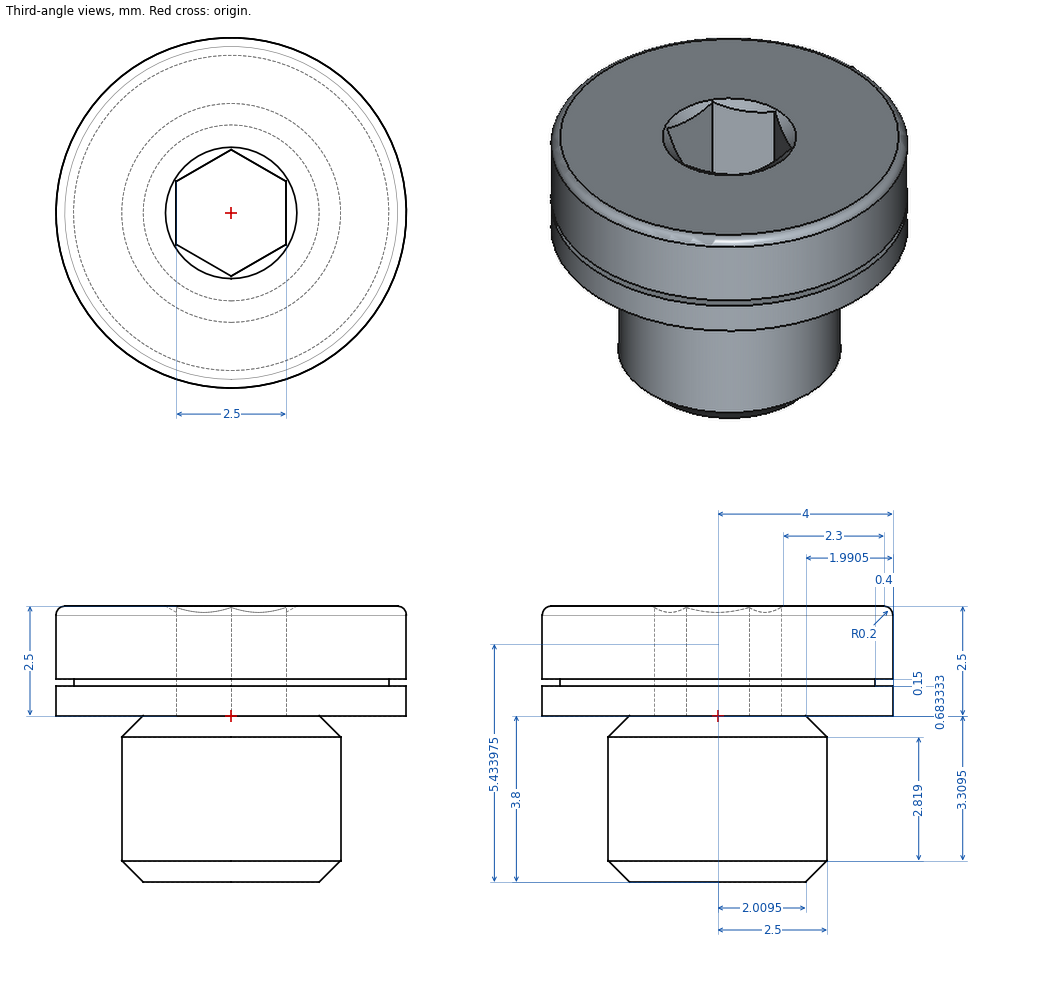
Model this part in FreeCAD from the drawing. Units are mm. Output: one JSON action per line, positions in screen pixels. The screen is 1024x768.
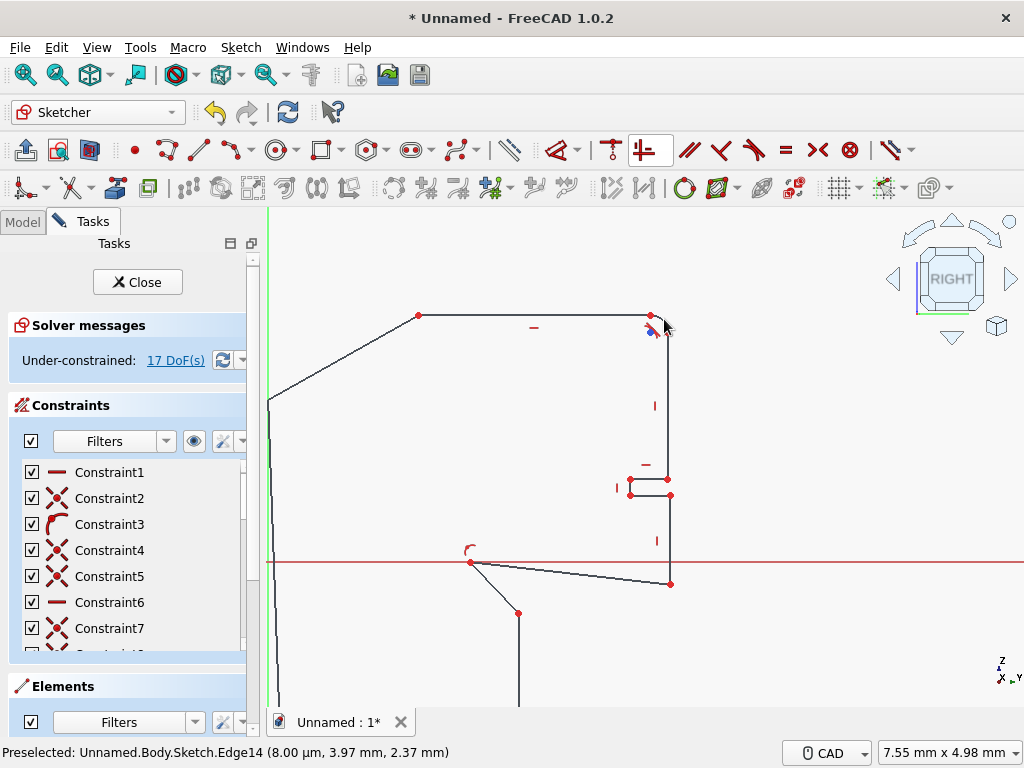
{"action": "scroll", "coordinate": [664, 318], "scroll_direction": "down", "scroll_amount": 4}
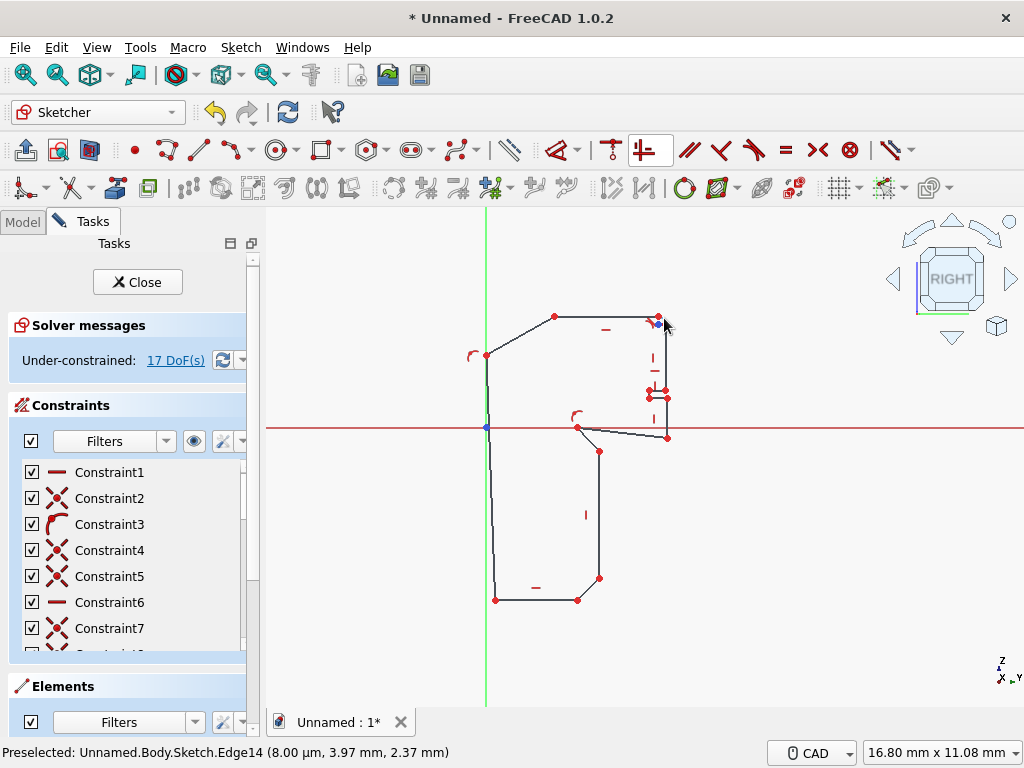
{"action": "scroll", "coordinate": [493, 527], "scroll_direction": "up", "scroll_amount": 5}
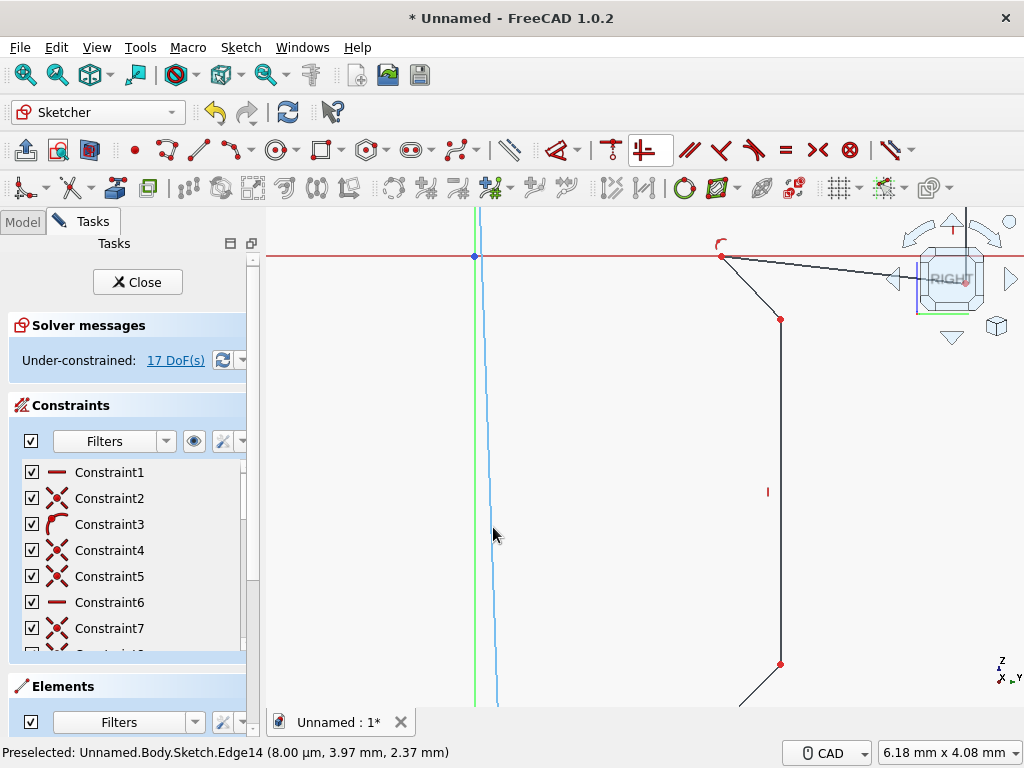
{"action": "left_click", "coordinate": [491, 525]}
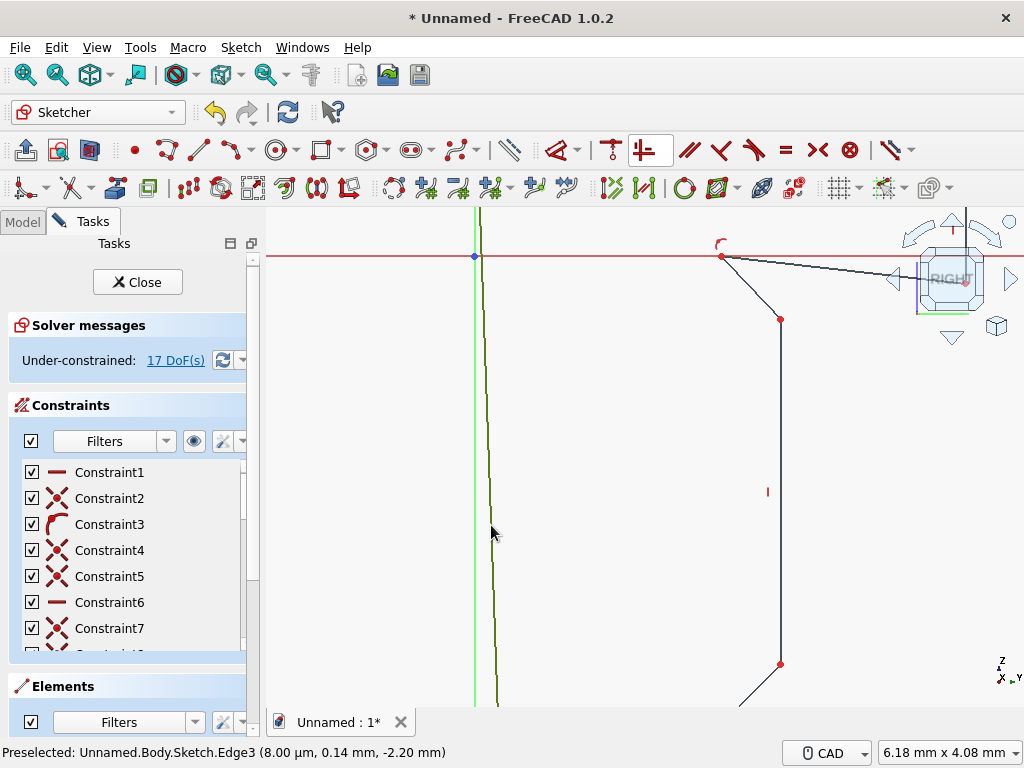
{"action": "left_click", "coordinate": [668, 150]}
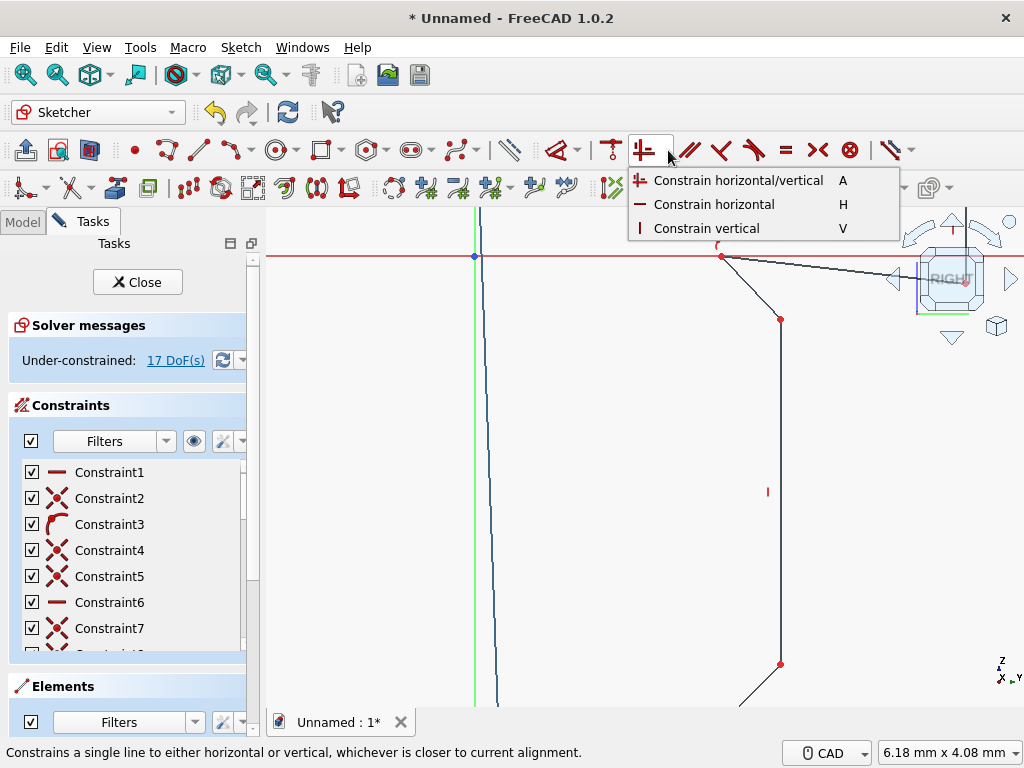
{"action": "left_click", "coordinate": [764, 228]}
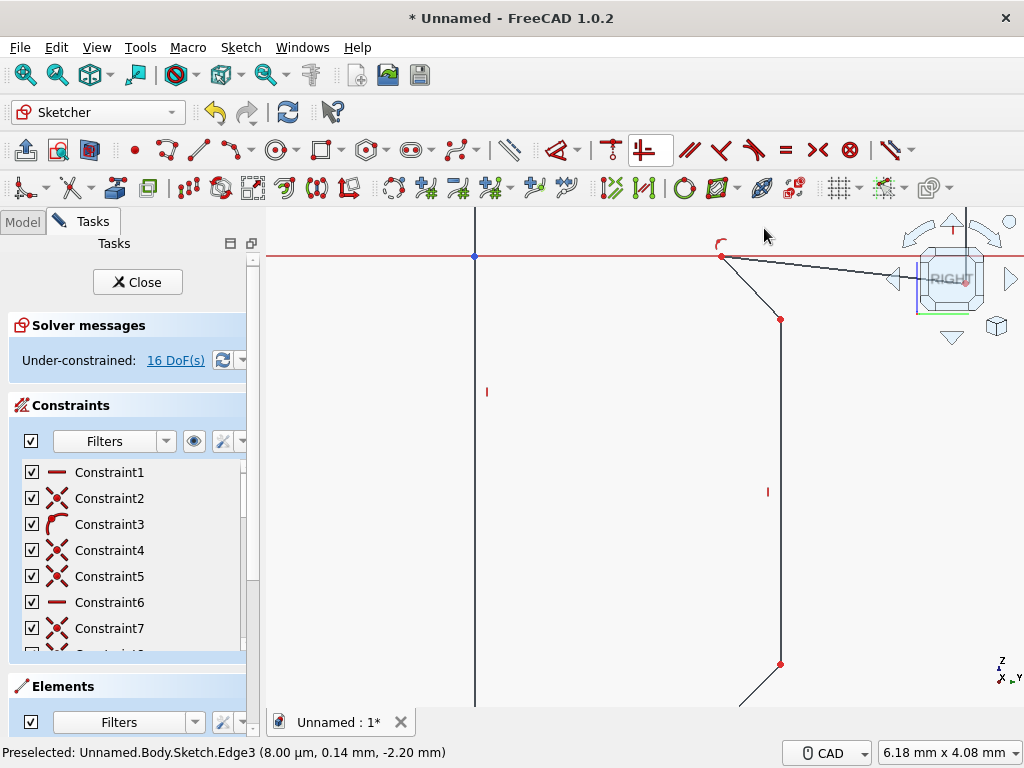
{"action": "scroll", "coordinate": [819, 267], "scroll_direction": "up", "scroll_amount": 2}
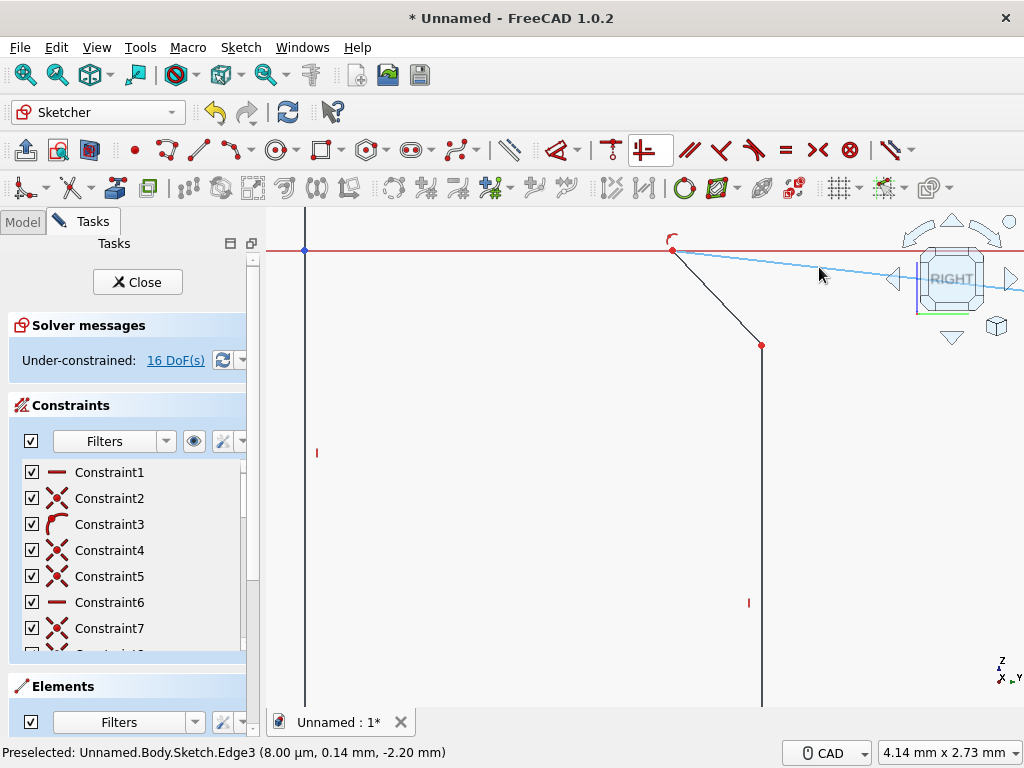
{"action": "left_click", "coordinate": [819, 268]}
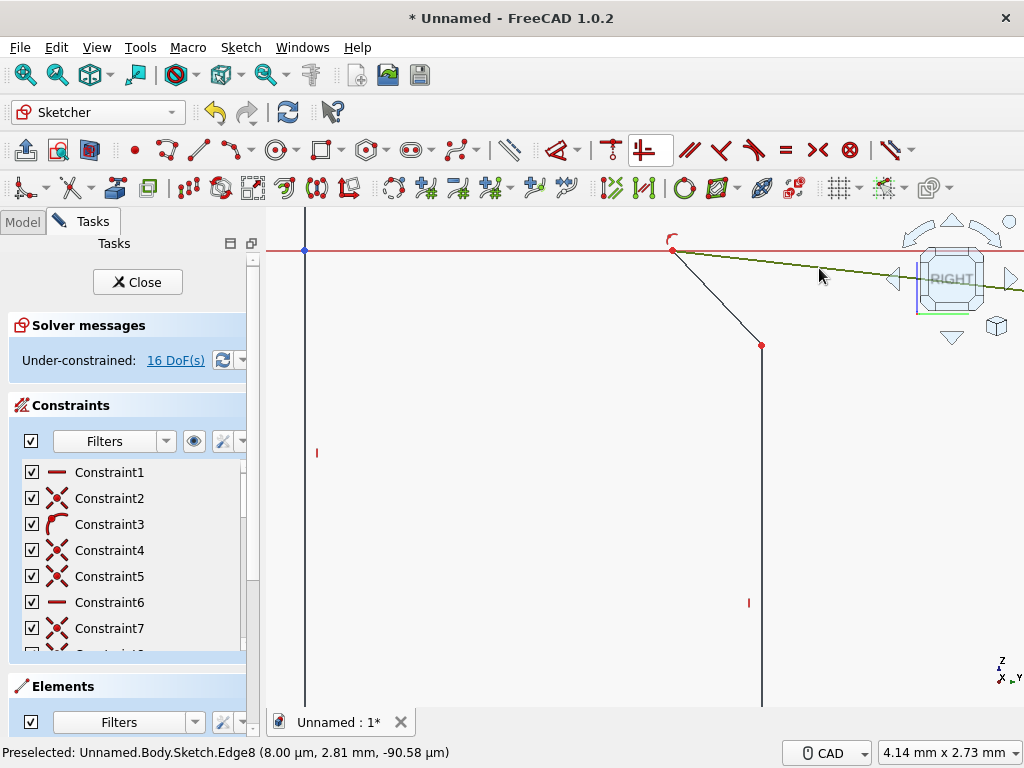
{"action": "key", "text": "h"}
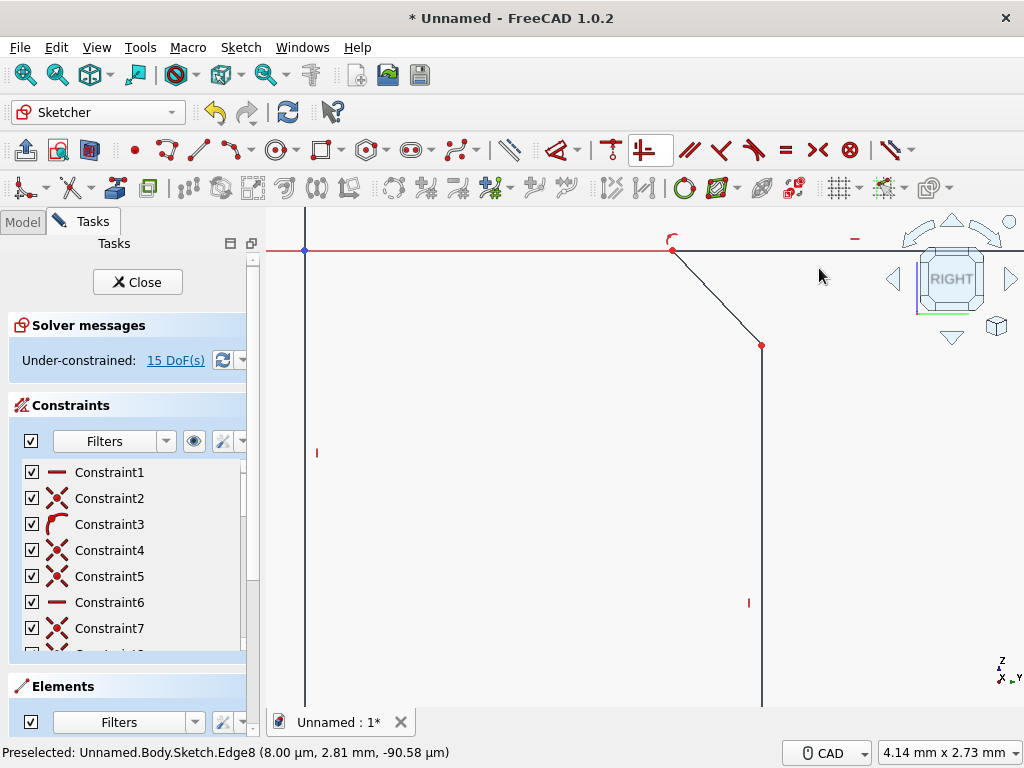
{"action": "key", "text": "d"}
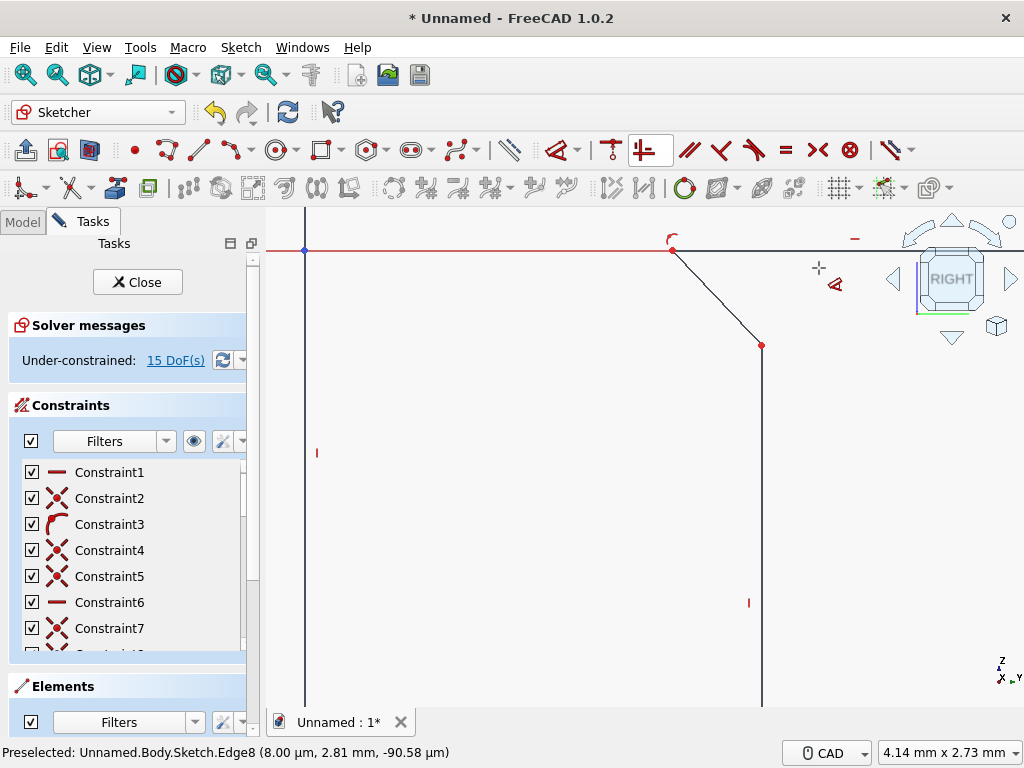
{"action": "scroll", "coordinate": [546, 485], "scroll_direction": "down", "scroll_amount": 7}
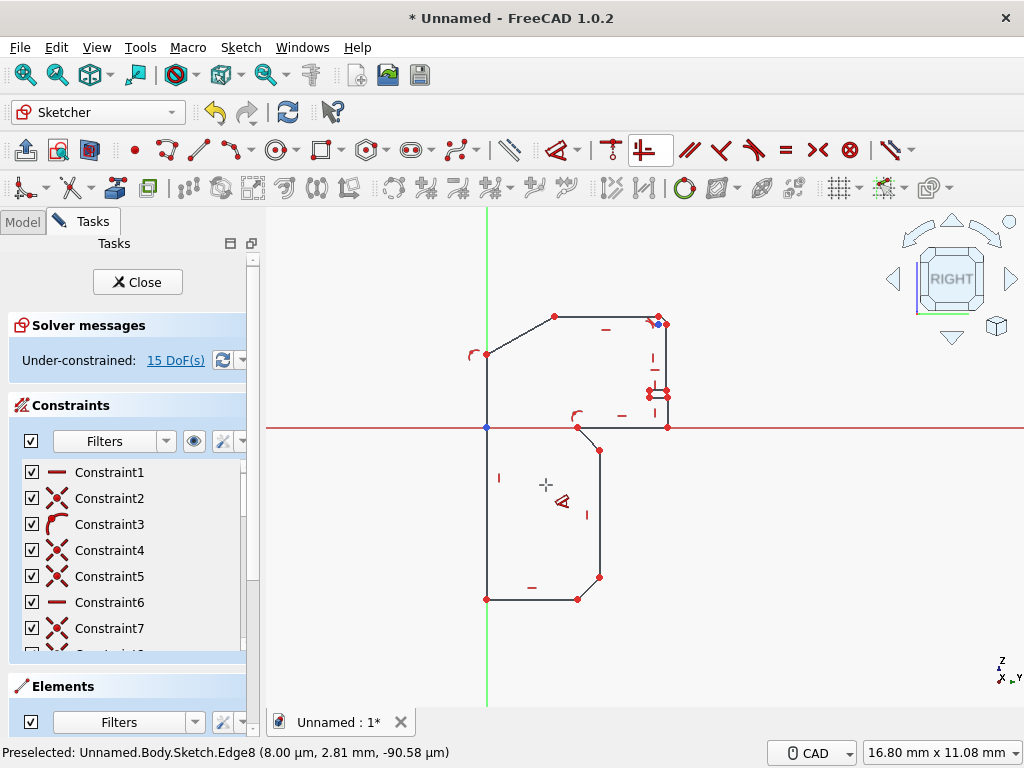
{"action": "scroll", "coordinate": [665, 321], "scroll_direction": "up", "scroll_amount": 8}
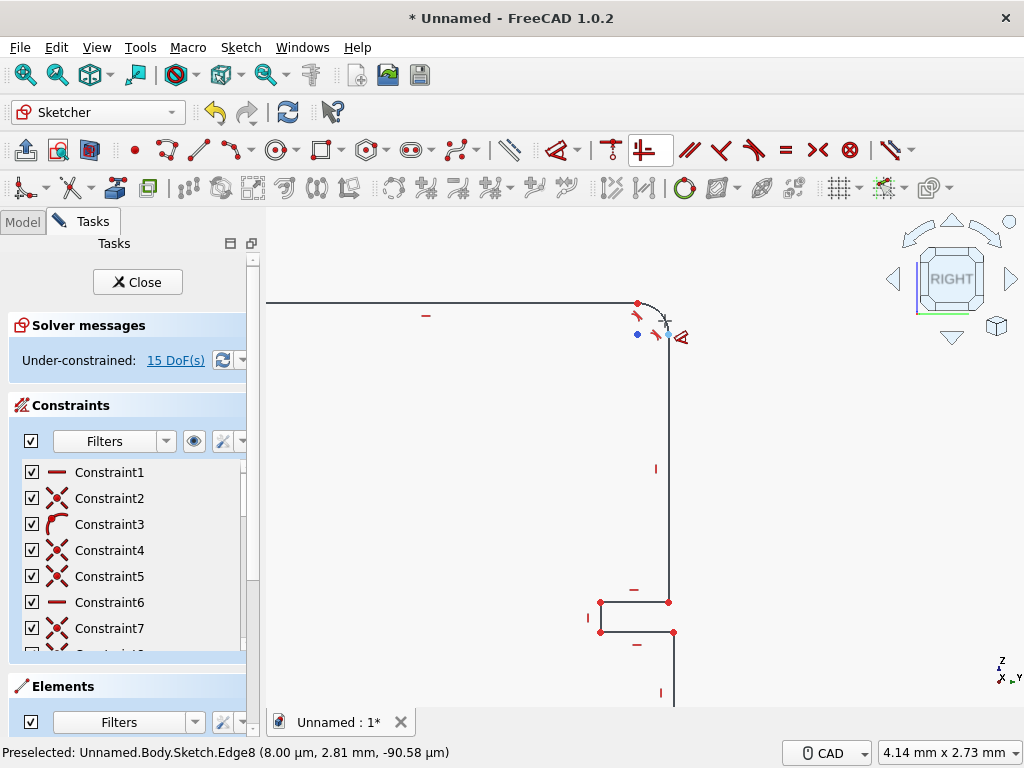
{"action": "left_click", "coordinate": [665, 320]}
{"action": "left_click", "coordinate": [693, 305]}